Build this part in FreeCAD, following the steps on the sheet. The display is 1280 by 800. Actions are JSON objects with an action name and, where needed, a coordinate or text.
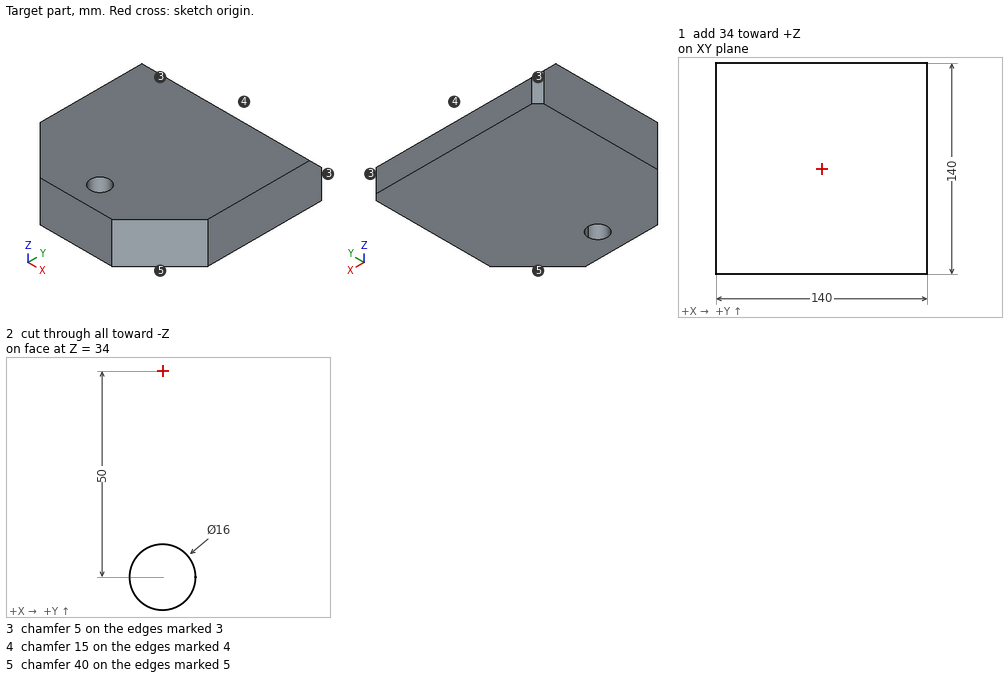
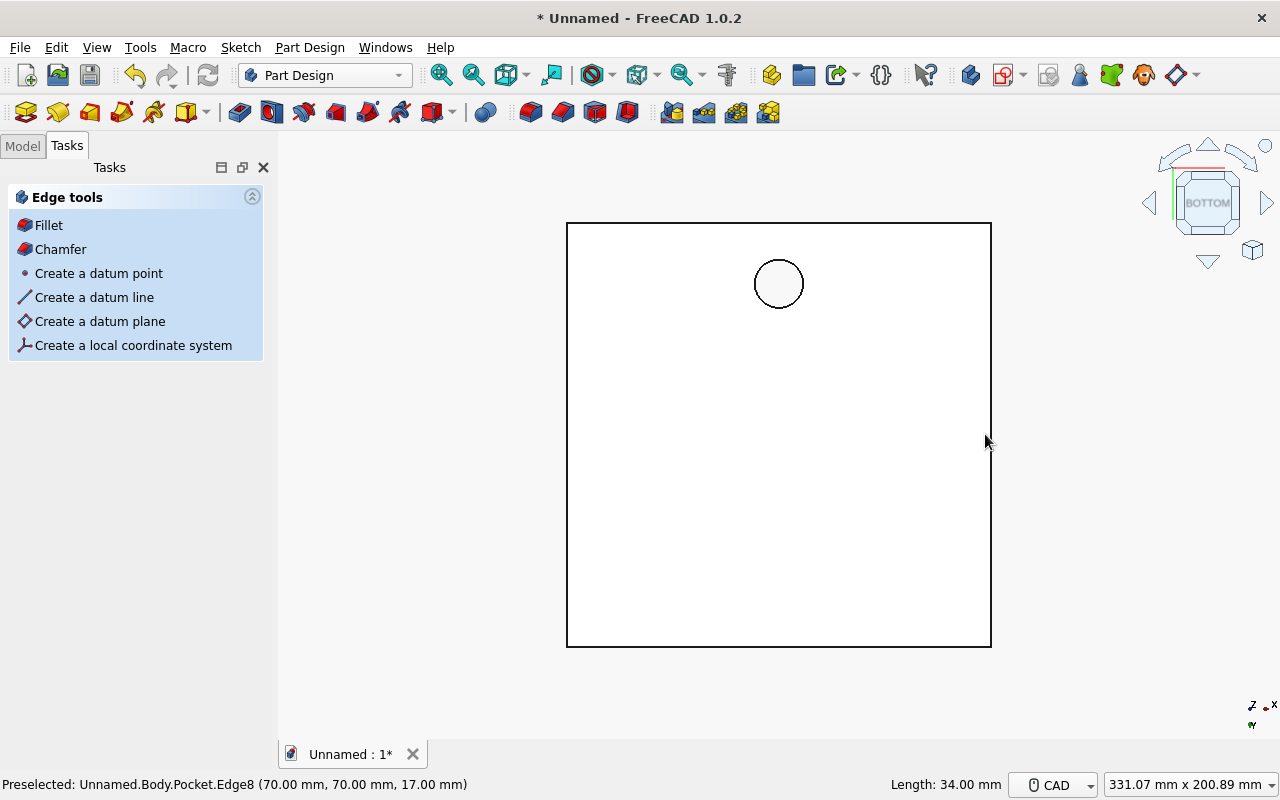
{"action": "key", "text": "4"}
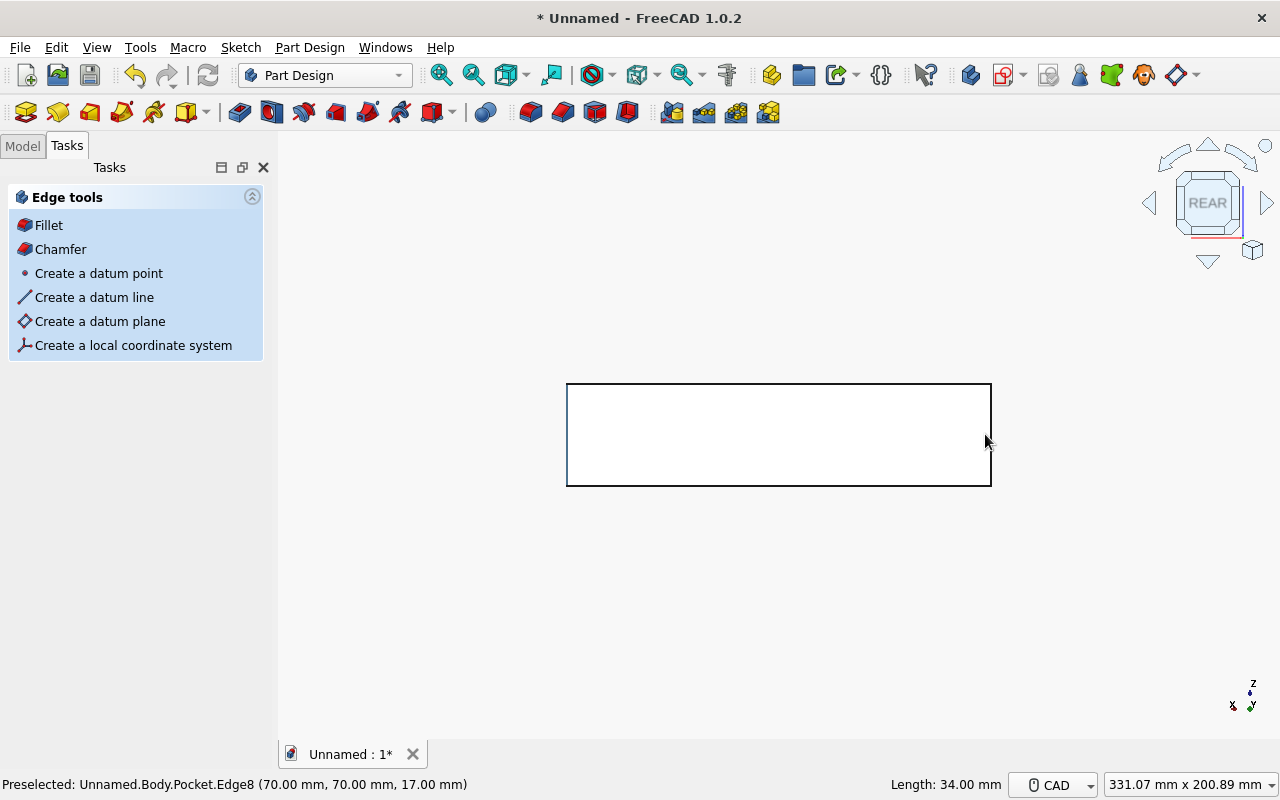
{"action": "left_click", "coordinate": [442, 76]}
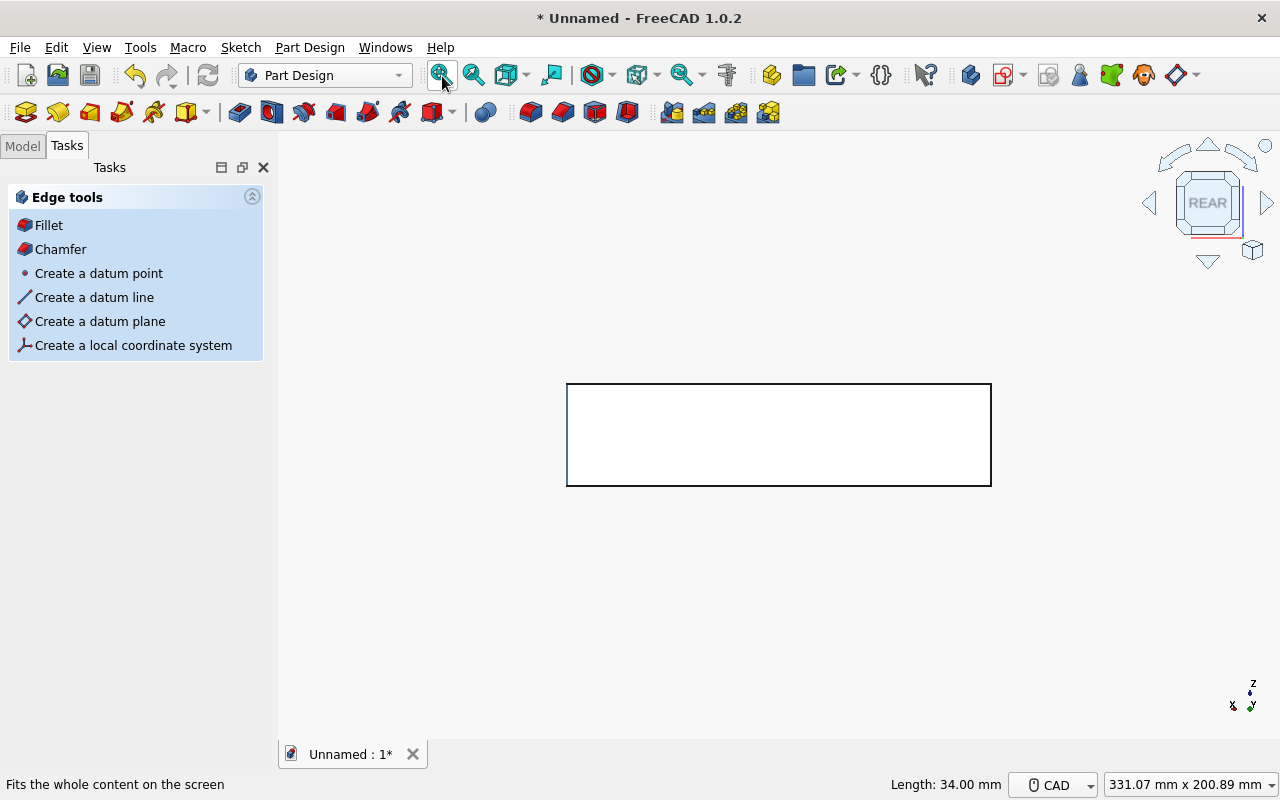
{"action": "left_click", "coordinate": [991, 434], "text": "ctrl"}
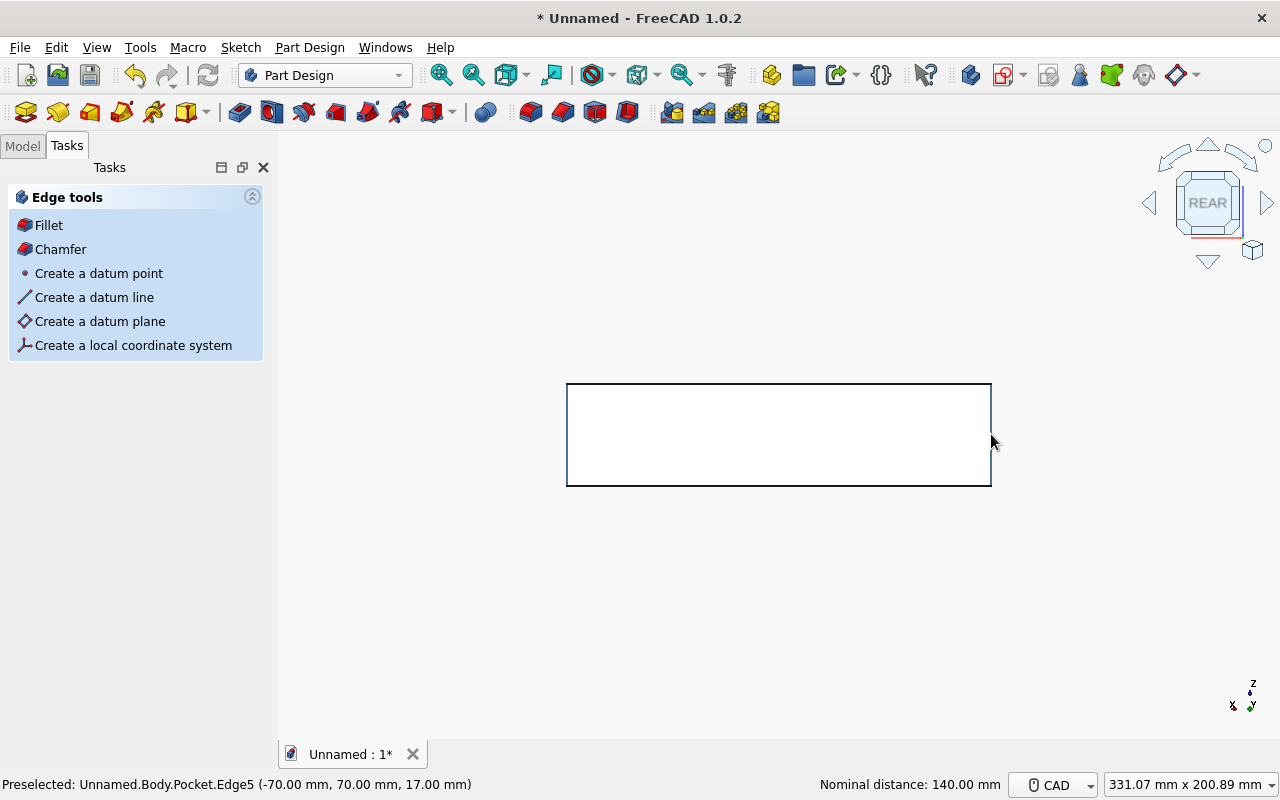
{"action": "left_click", "coordinate": [564, 112]}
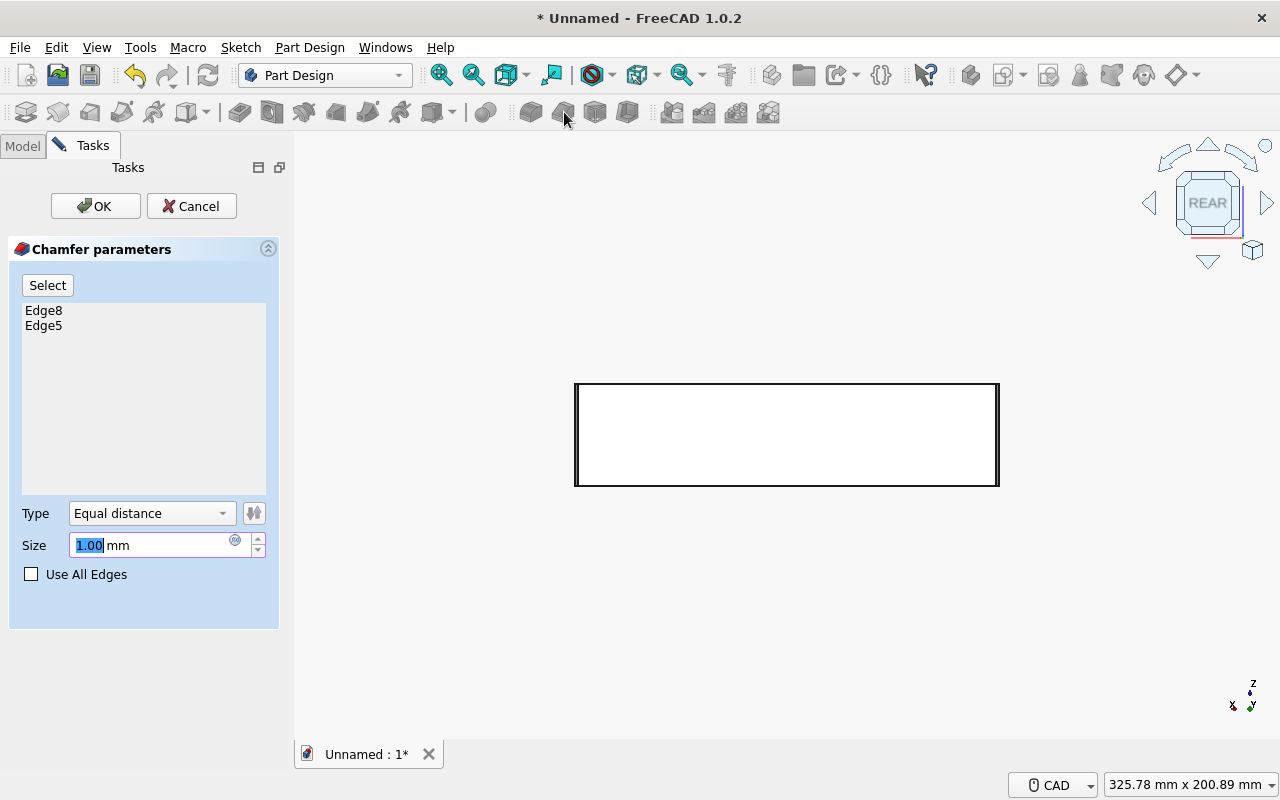
{"action": "type", "text": "5"}
{"action": "key", "text": "Tab"}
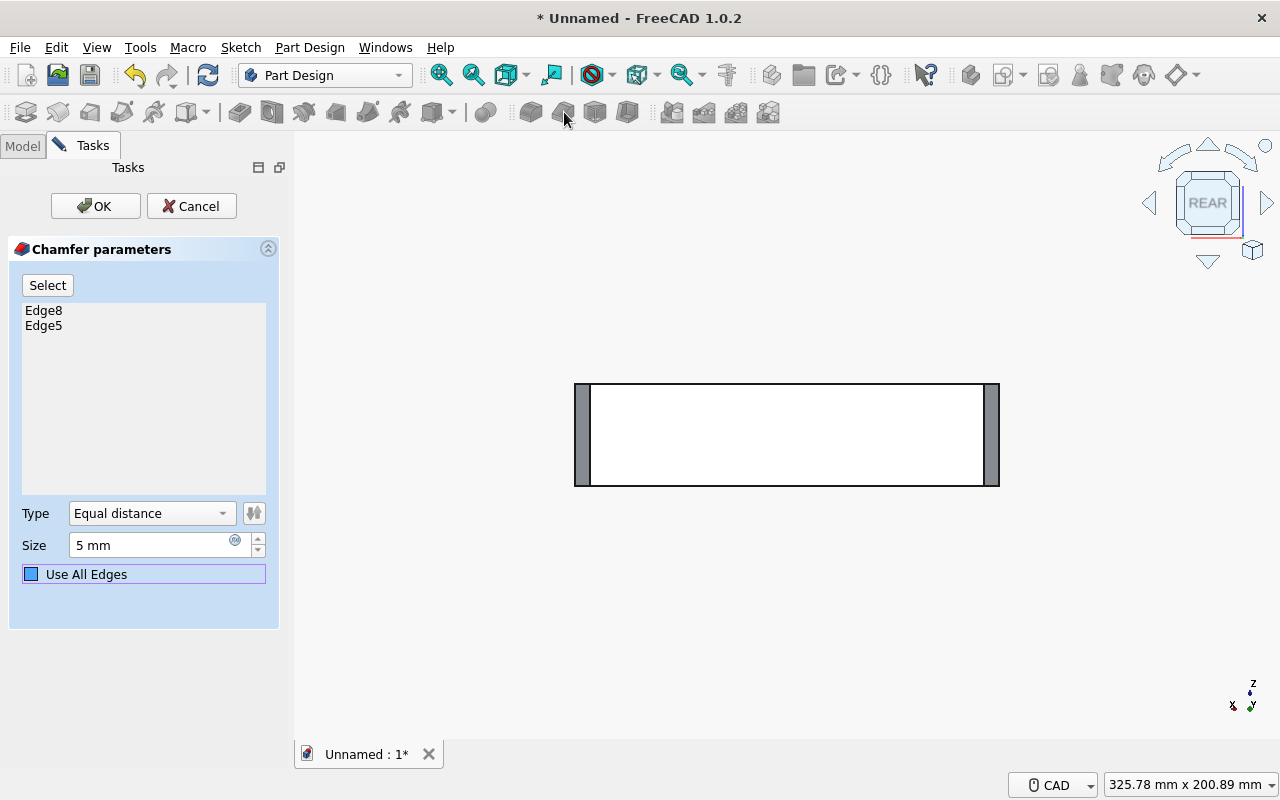
{"action": "left_click", "coordinate": [96, 206]}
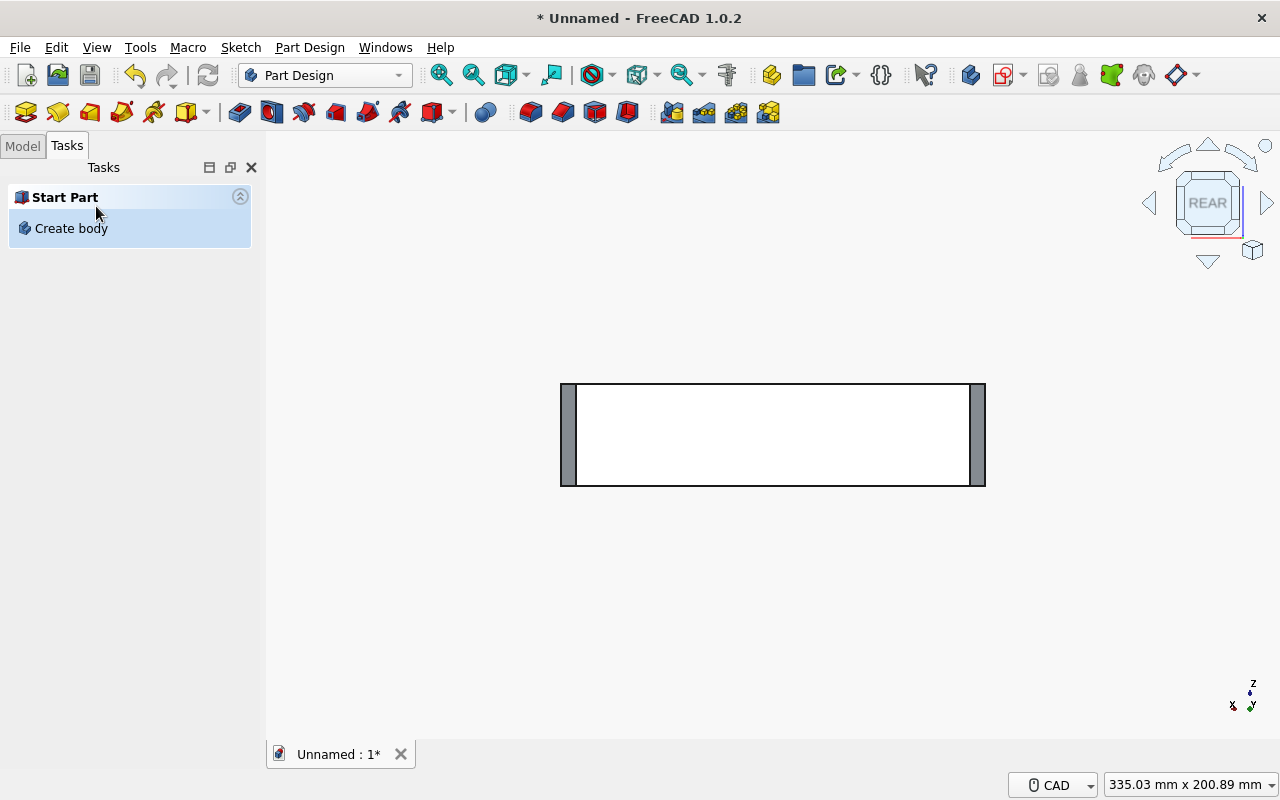
{"action": "key", "text": "v f"}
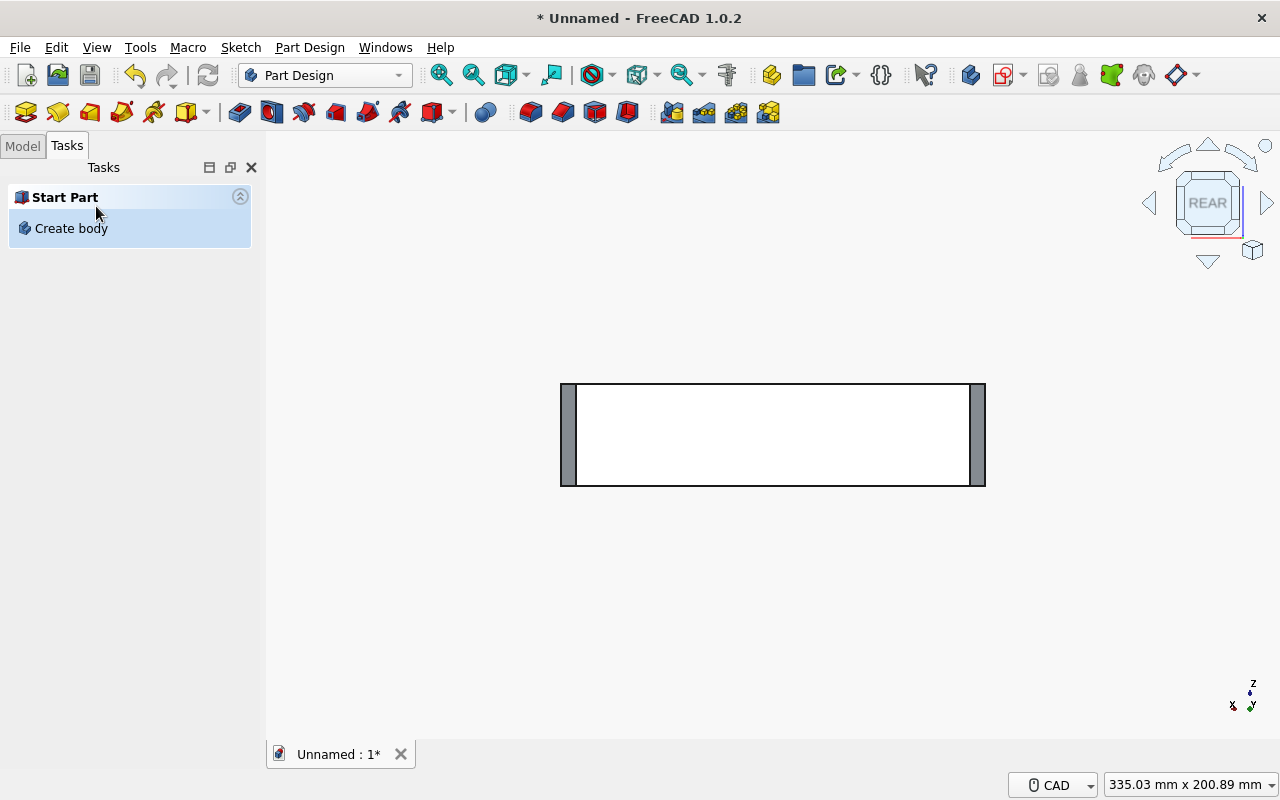
{"action": "left_click", "coordinate": [773, 383]}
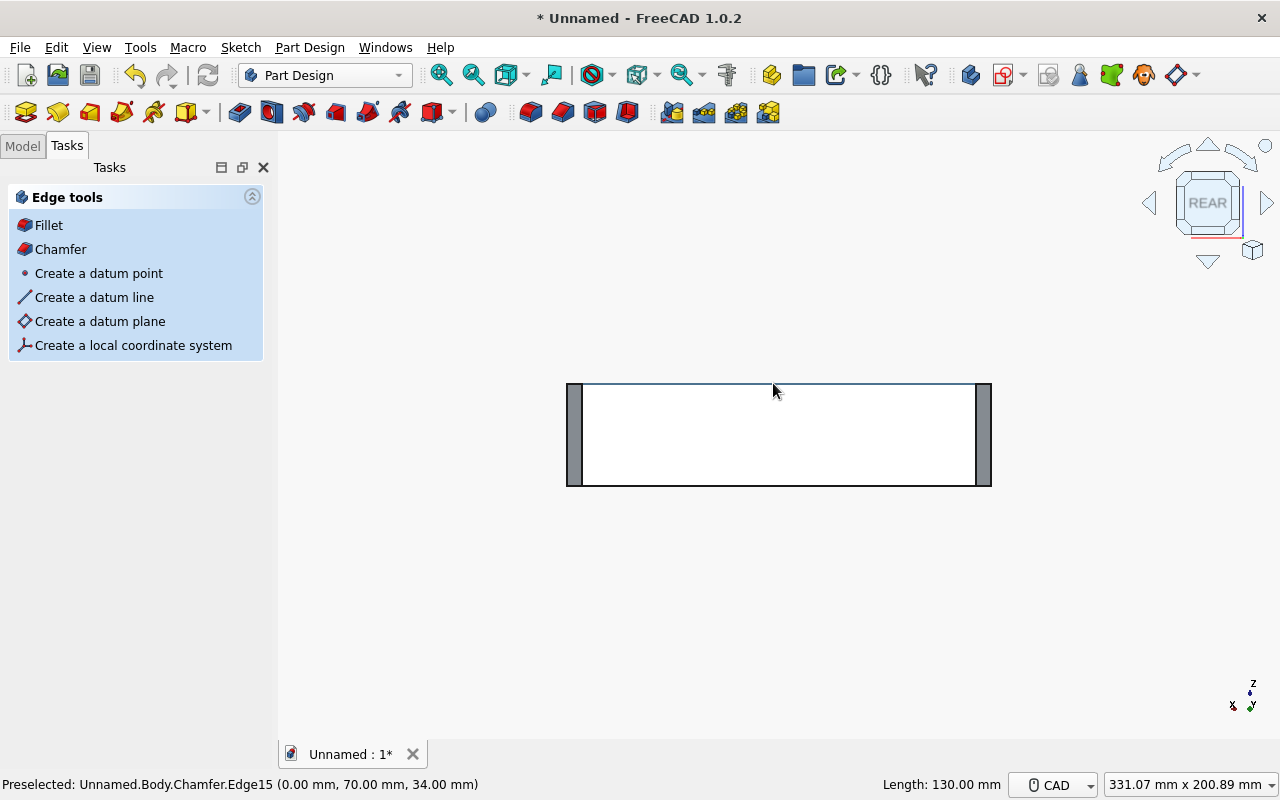
{"action": "left_click", "coordinate": [564, 112]}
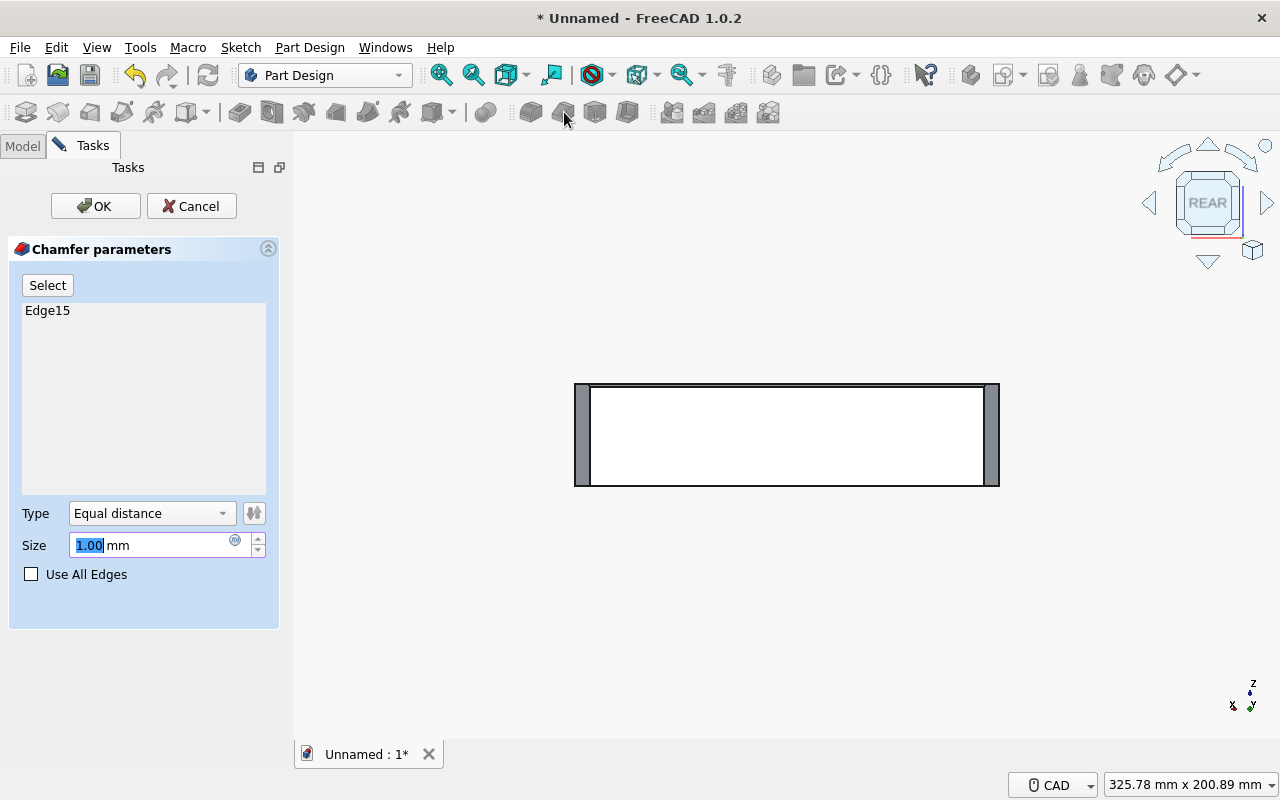
{"action": "type", "text": "15"}
{"action": "key", "text": "Tab"}